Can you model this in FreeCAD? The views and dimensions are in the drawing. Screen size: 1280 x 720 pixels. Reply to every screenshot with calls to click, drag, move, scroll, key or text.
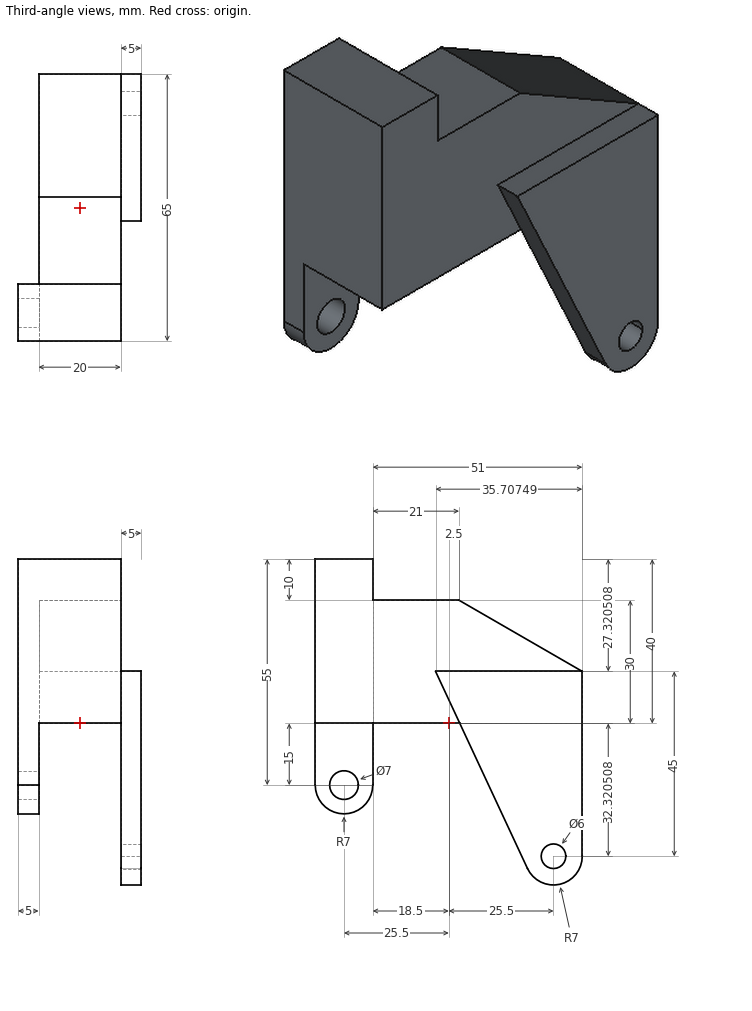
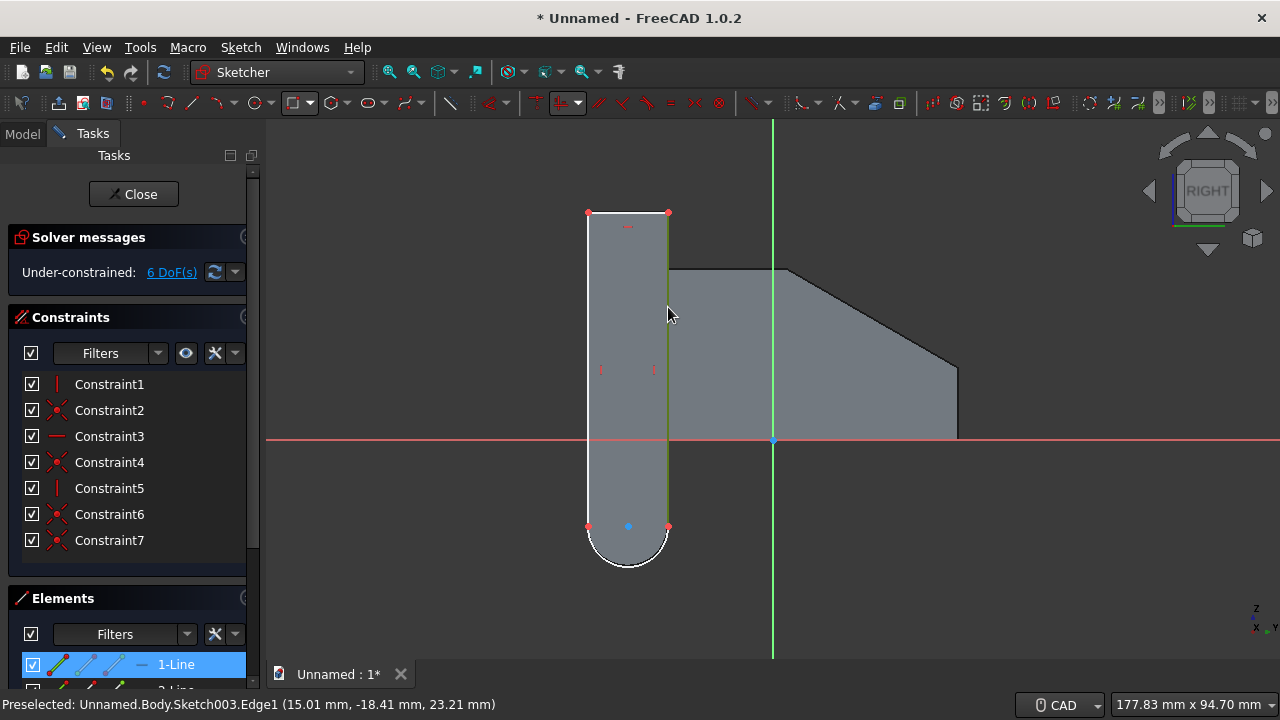
click(604, 559)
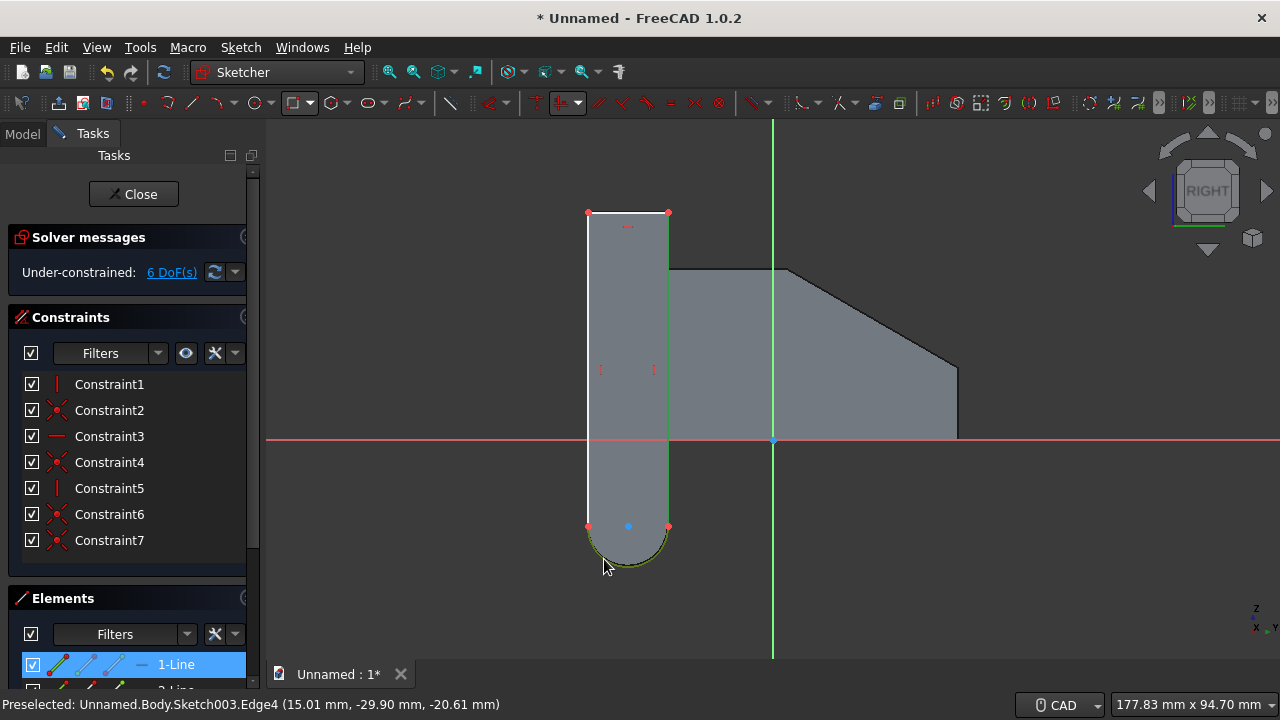
key(t)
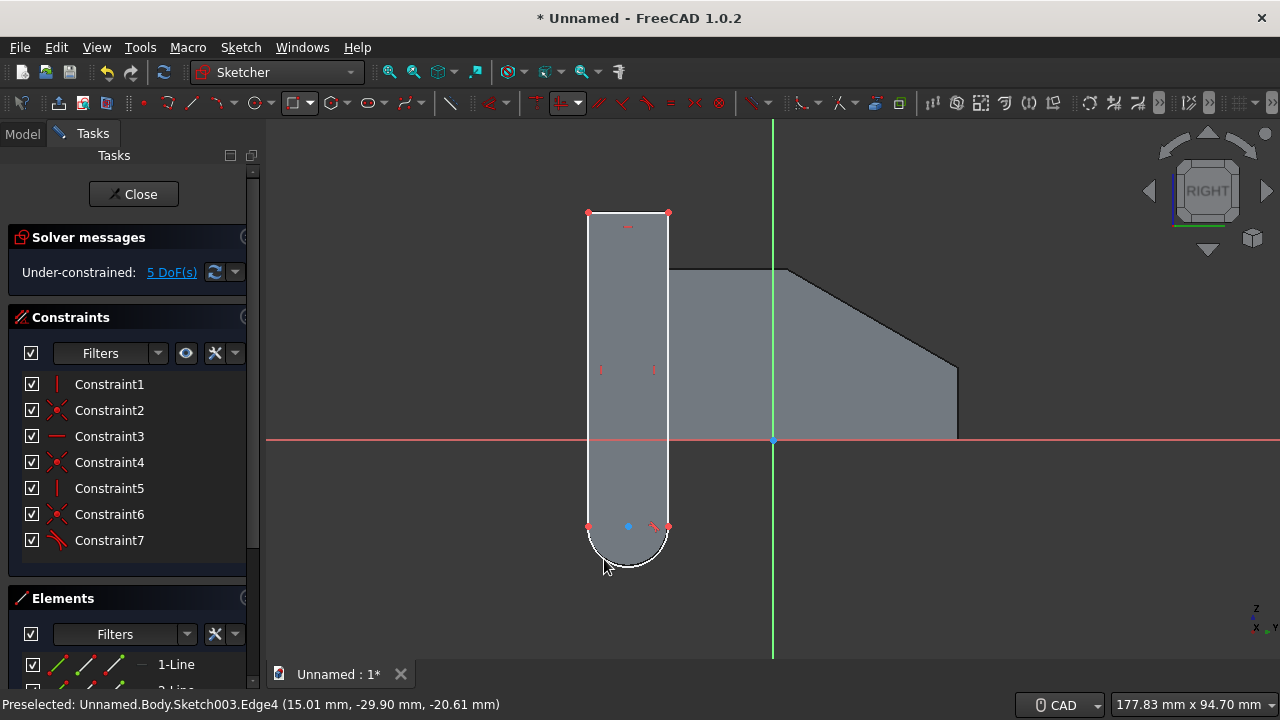
click(588, 307)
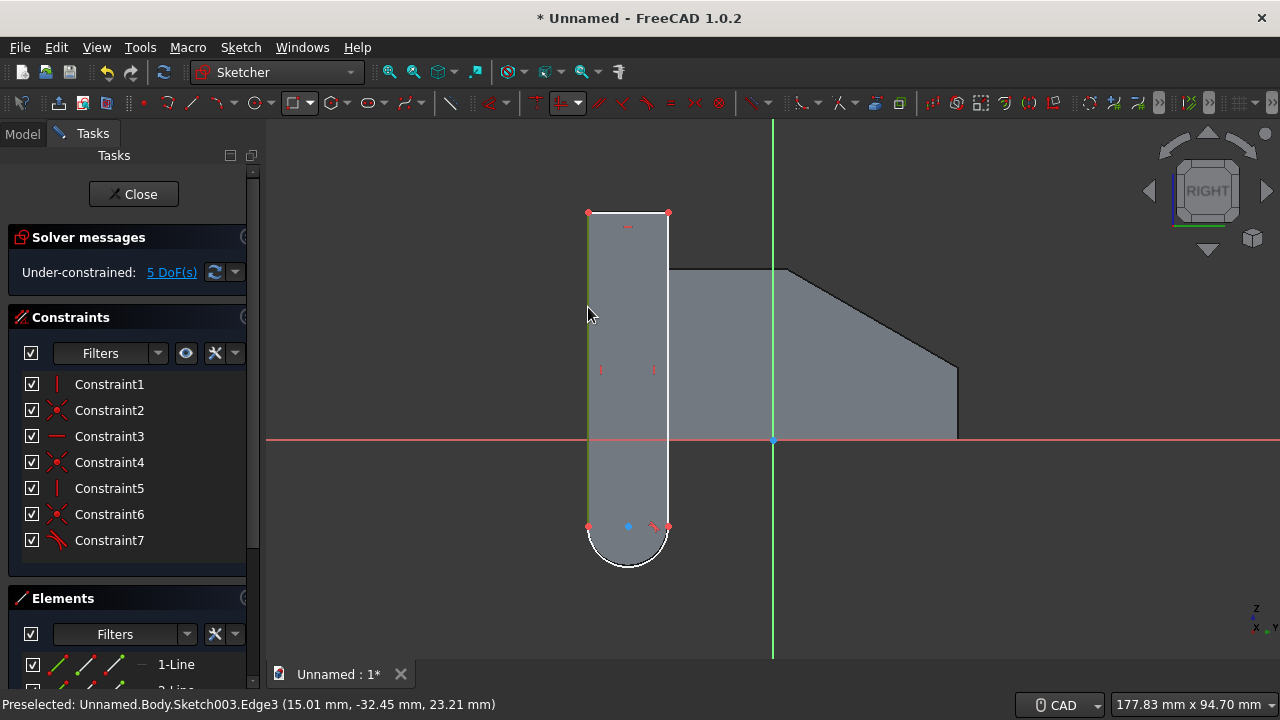
click(604, 559)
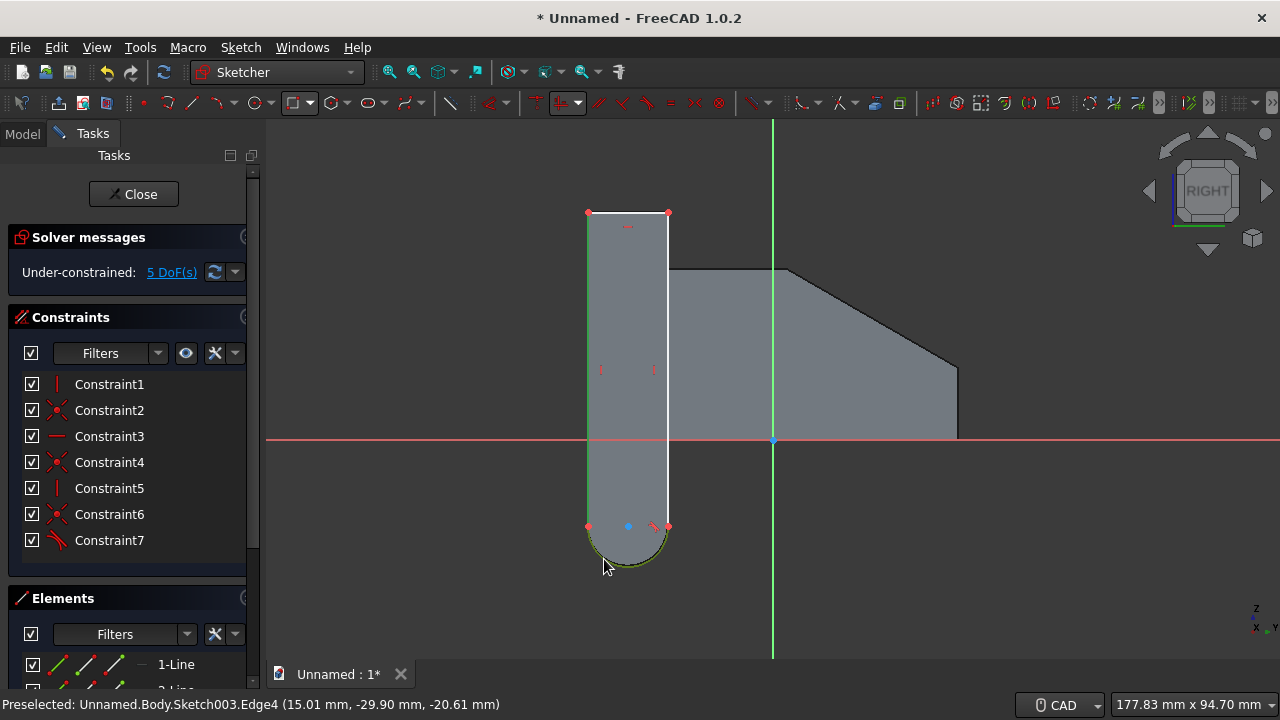
key(t)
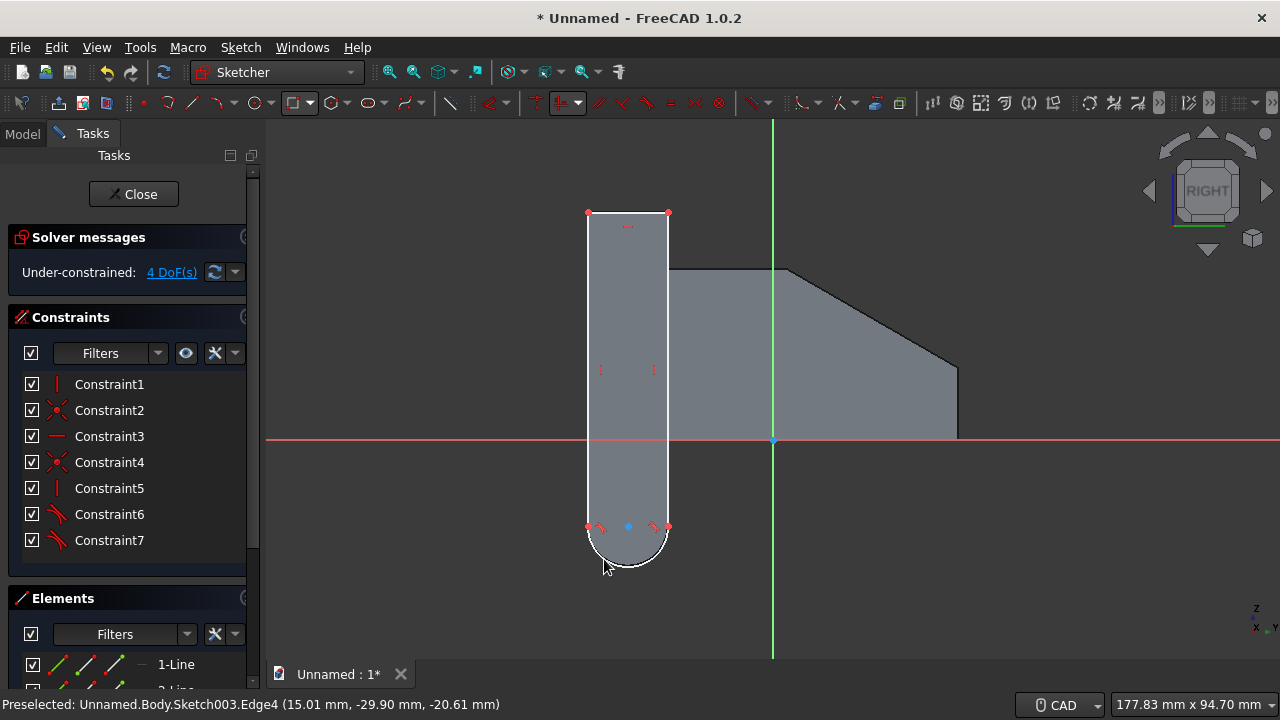
key(d)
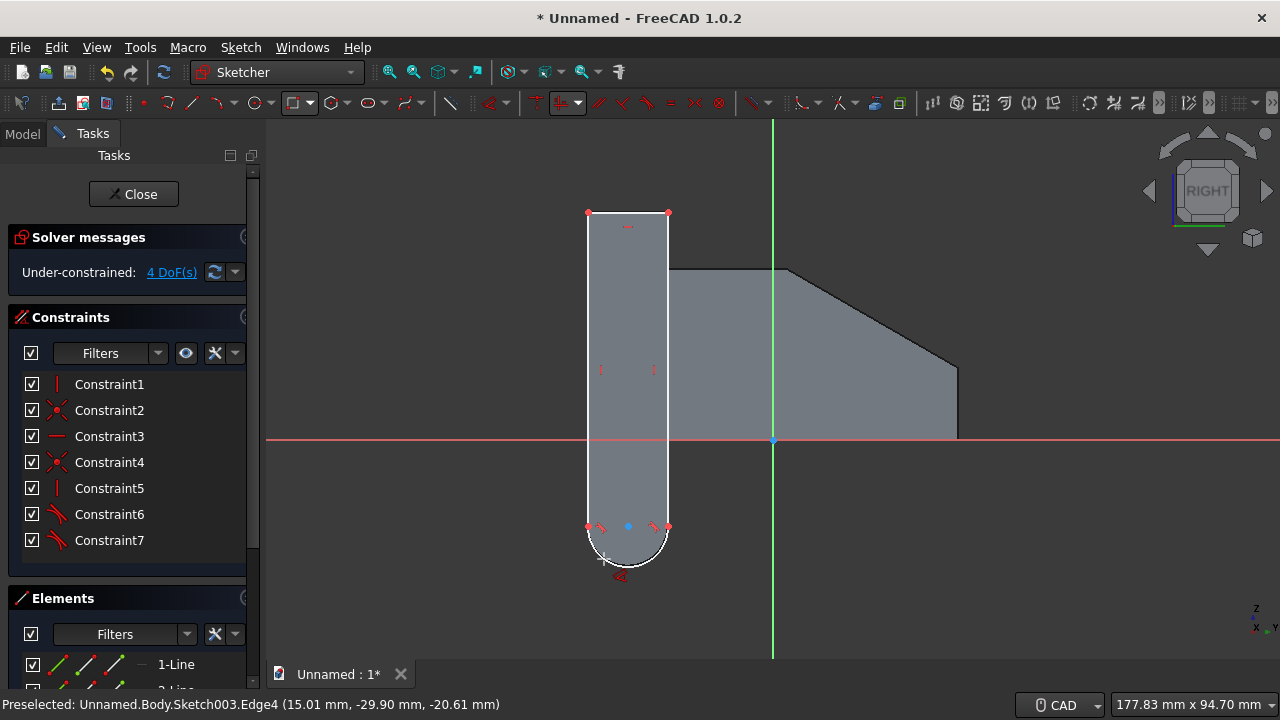
click(604, 559)
click(585, 585)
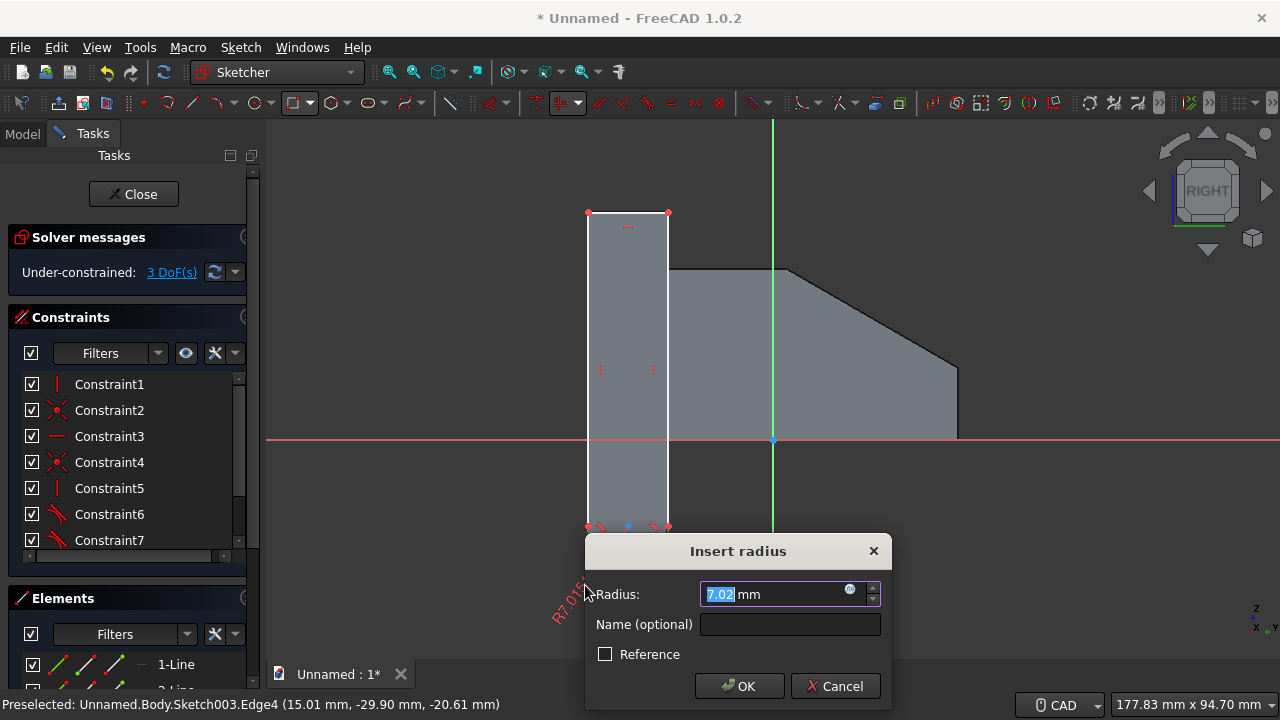
text(7)
key(Return)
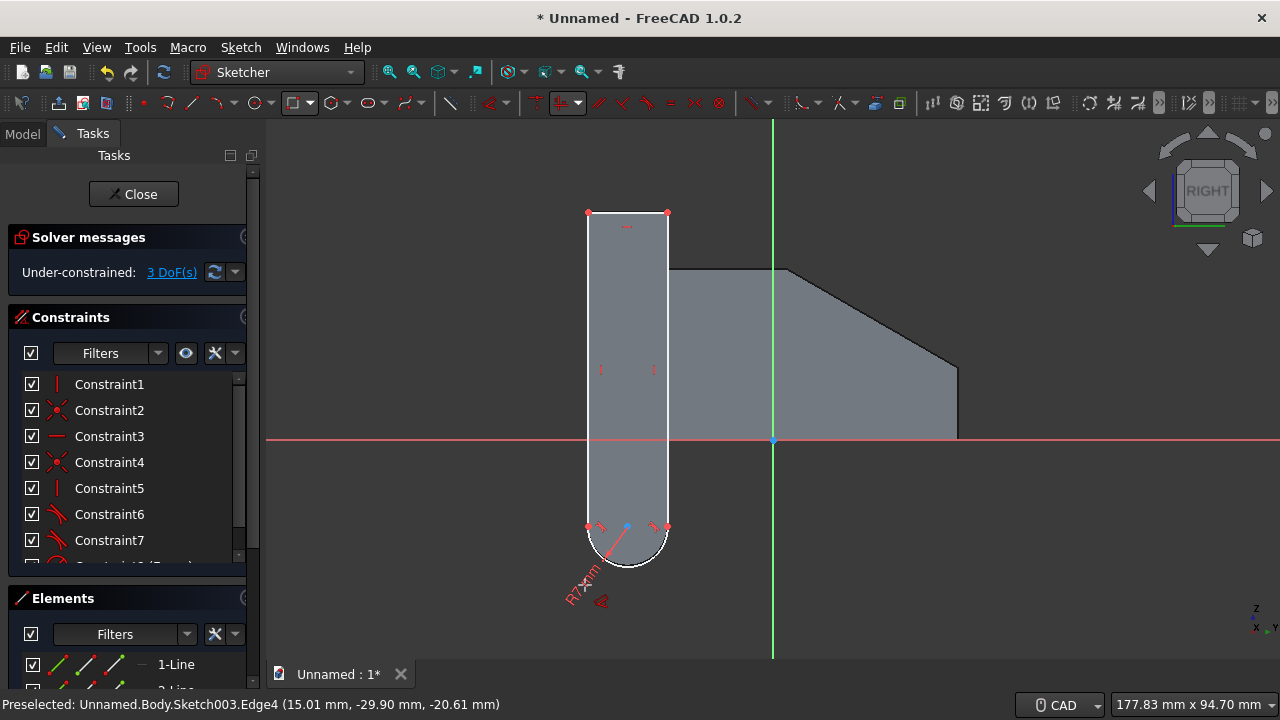
click(668, 307)
click(634, 370)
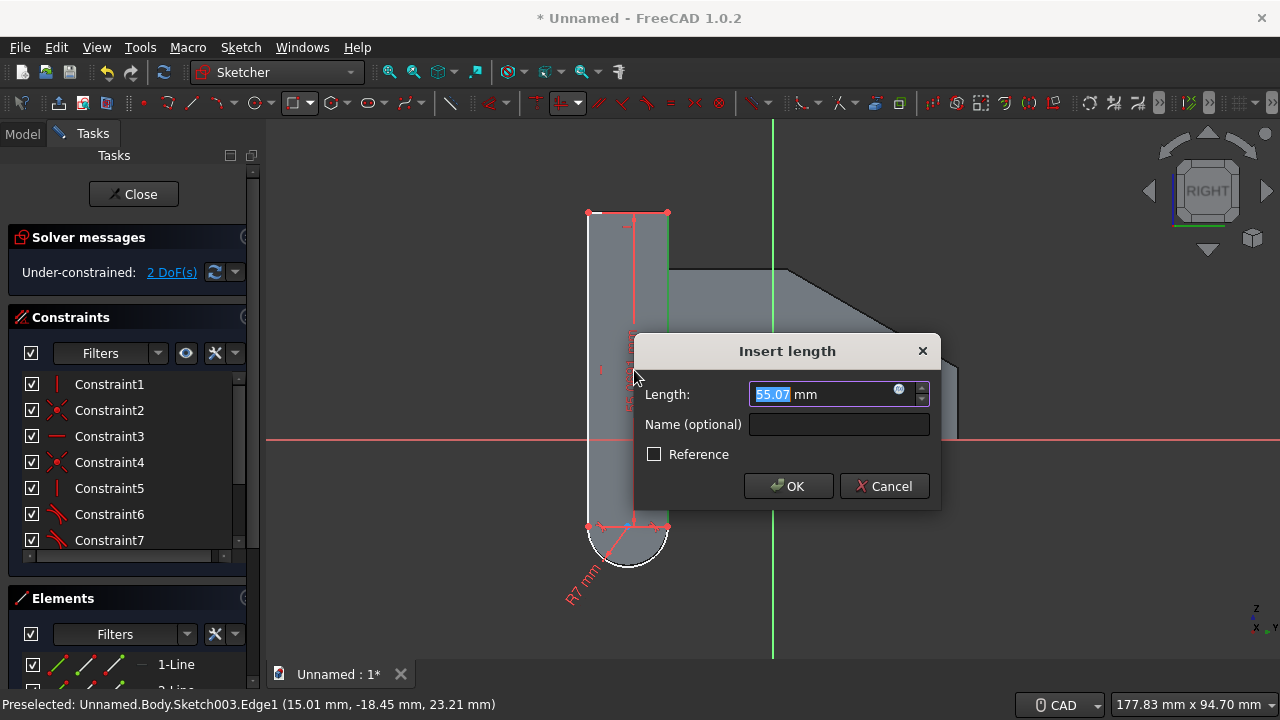
text(55)
key(Return)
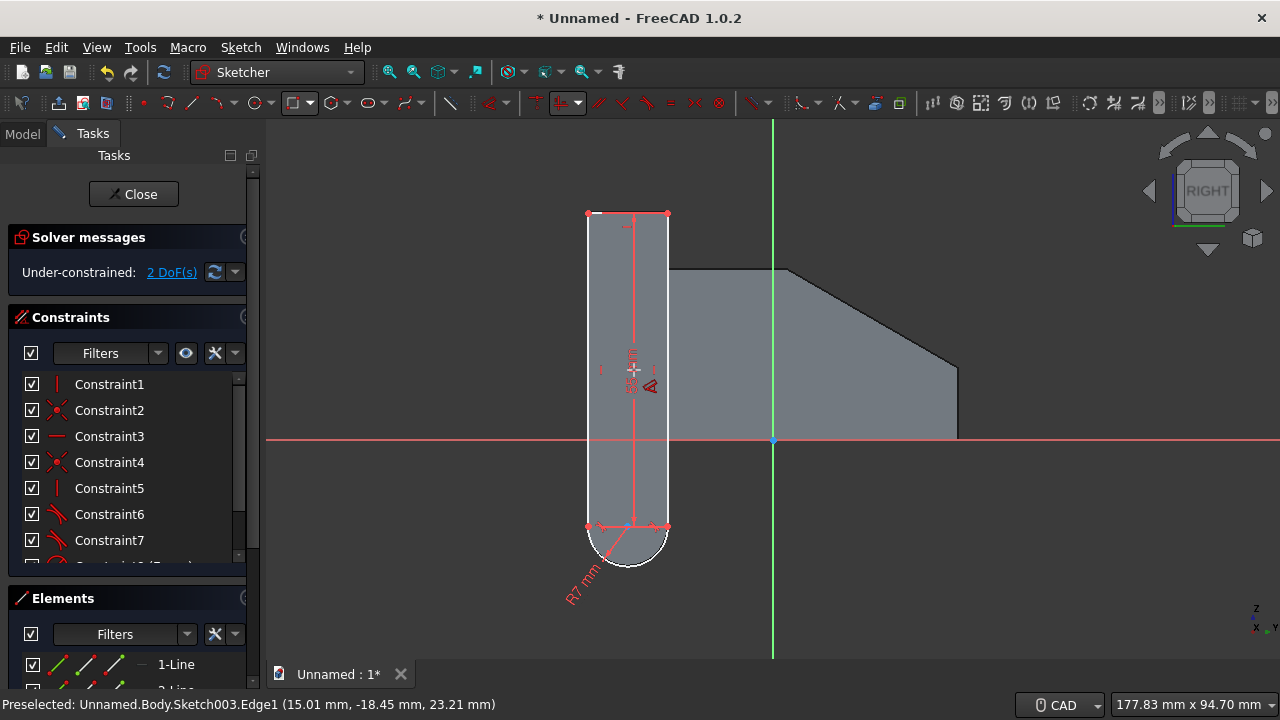
click(668, 527)
click(807, 483)